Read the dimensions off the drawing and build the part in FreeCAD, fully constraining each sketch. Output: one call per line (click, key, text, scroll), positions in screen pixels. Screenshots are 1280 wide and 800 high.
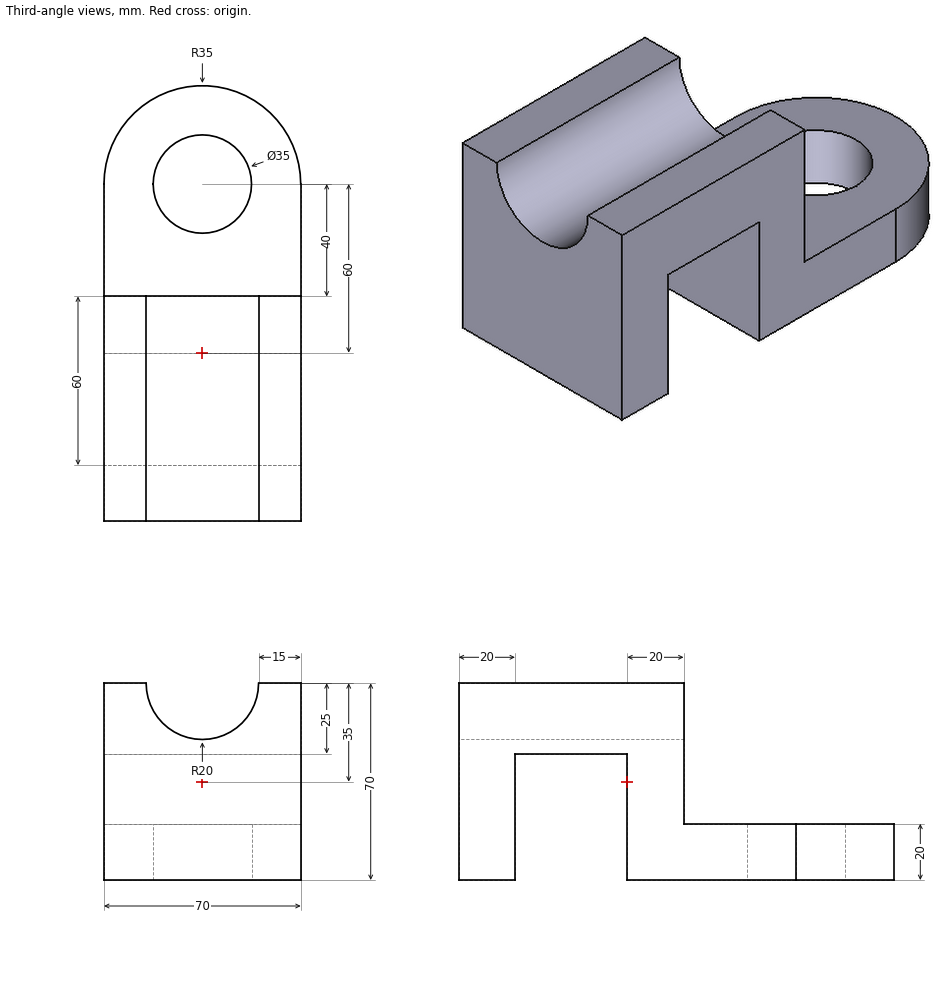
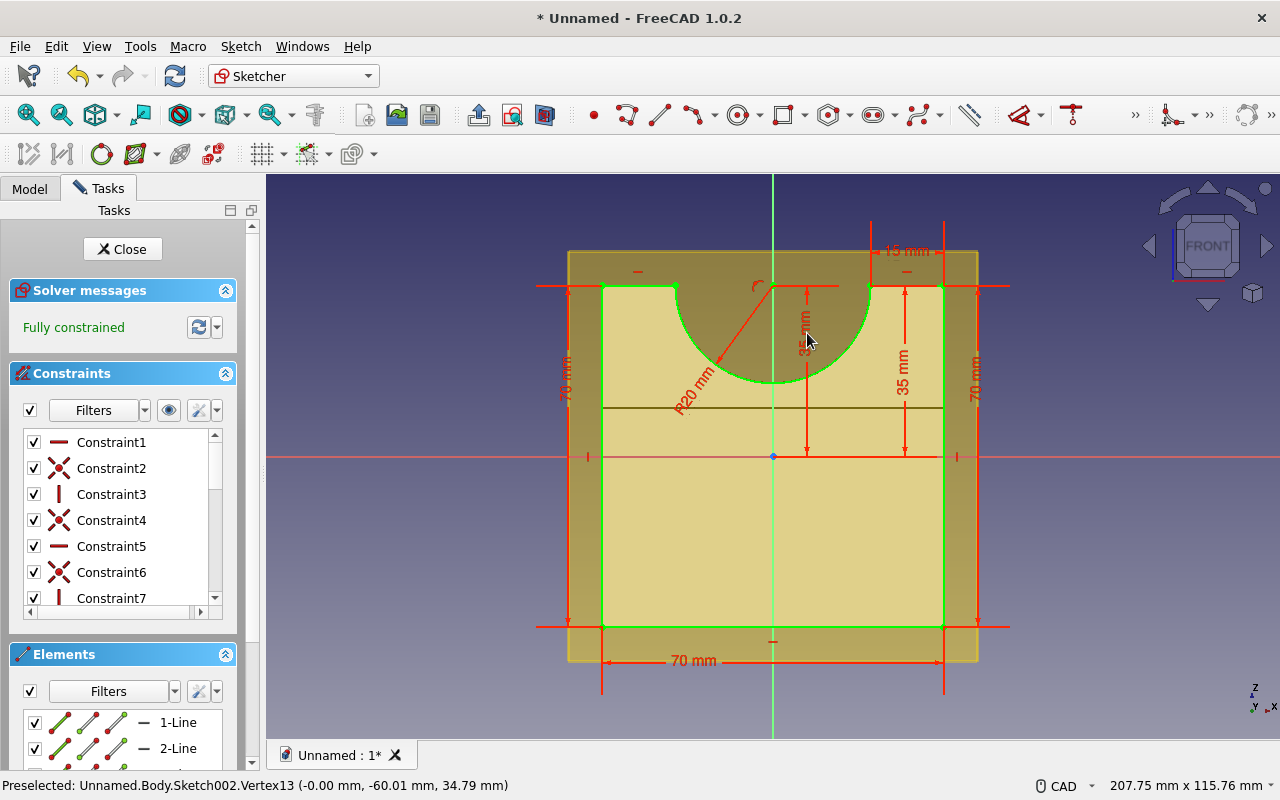
click(123, 249)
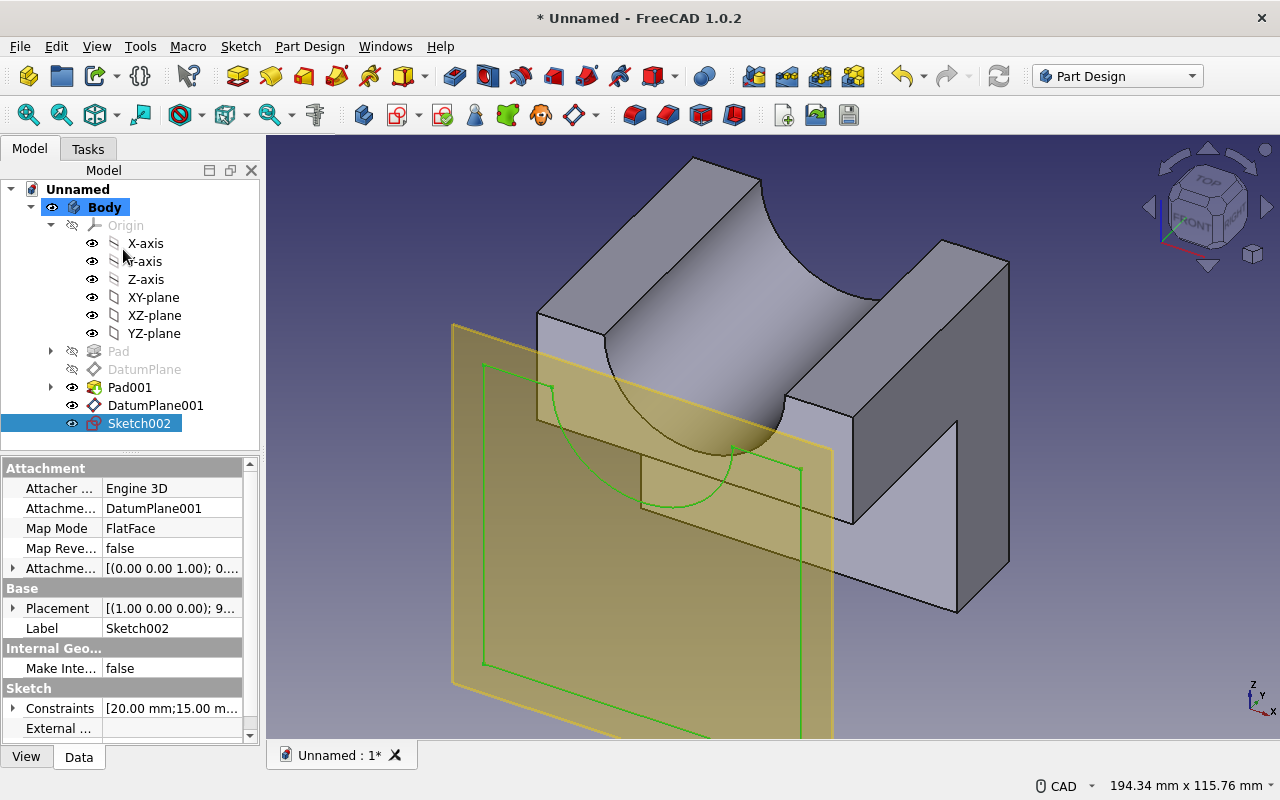
click(238, 76)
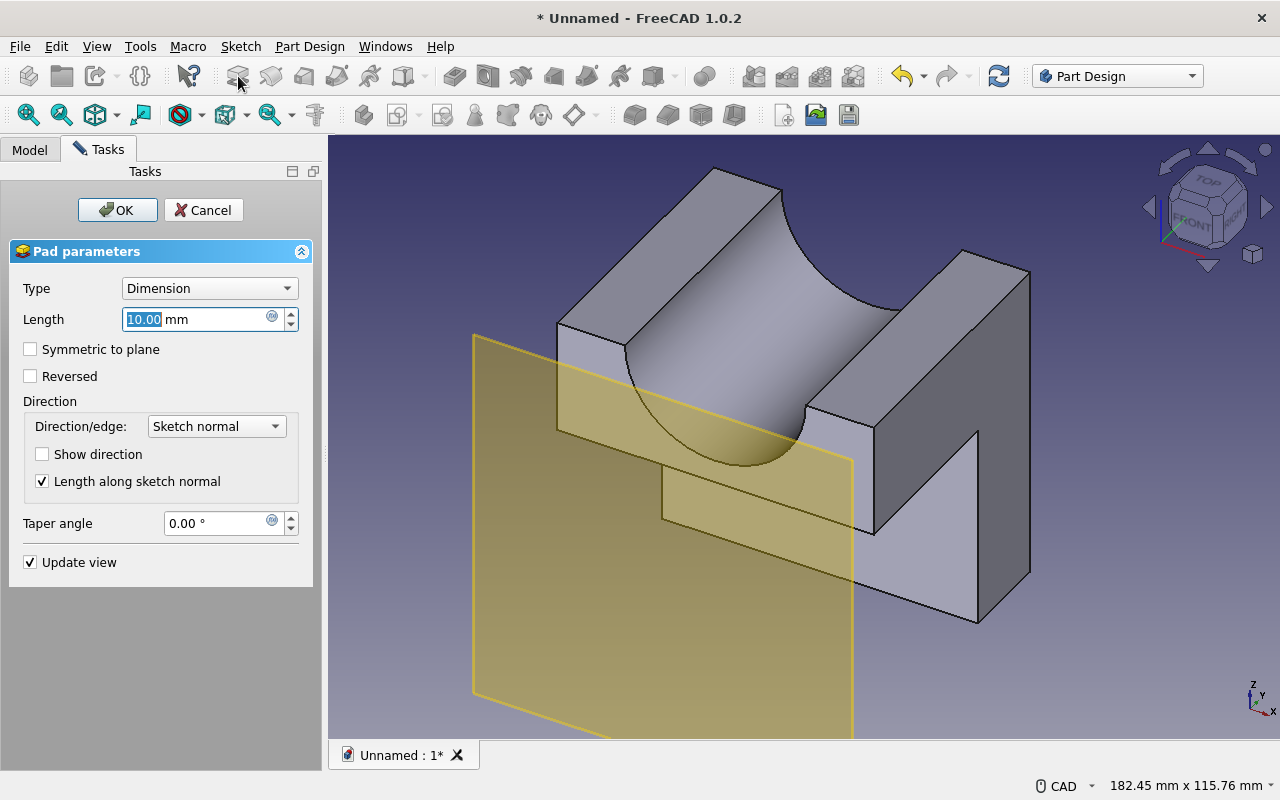
text(20)
key(Tab)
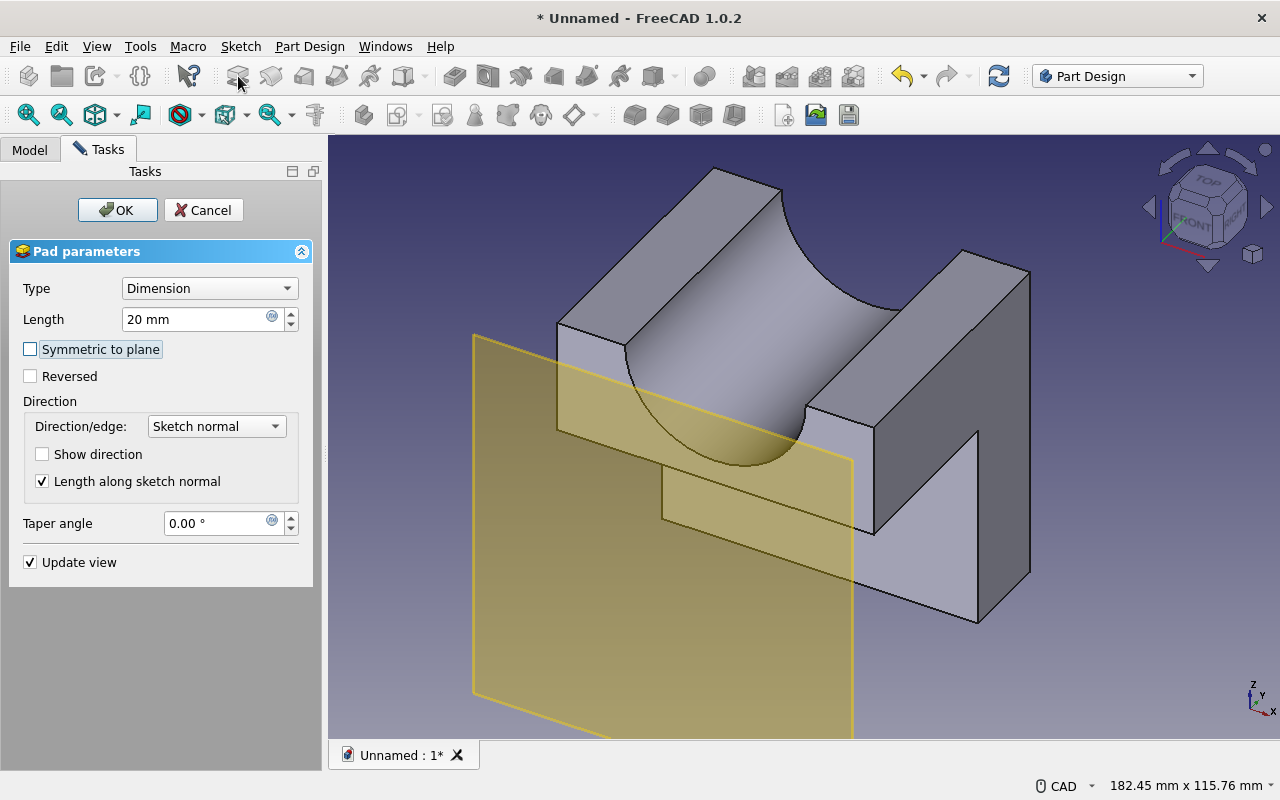
click(31, 376)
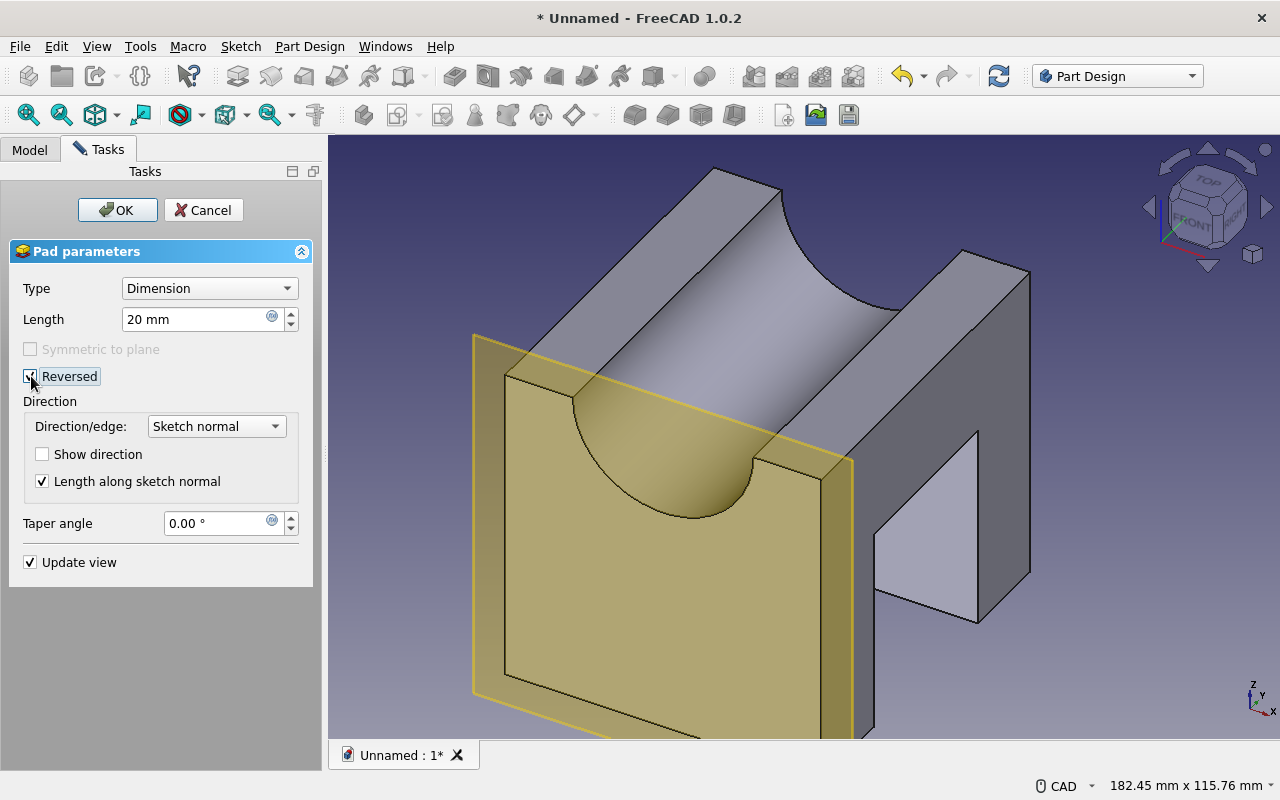
click(118, 210)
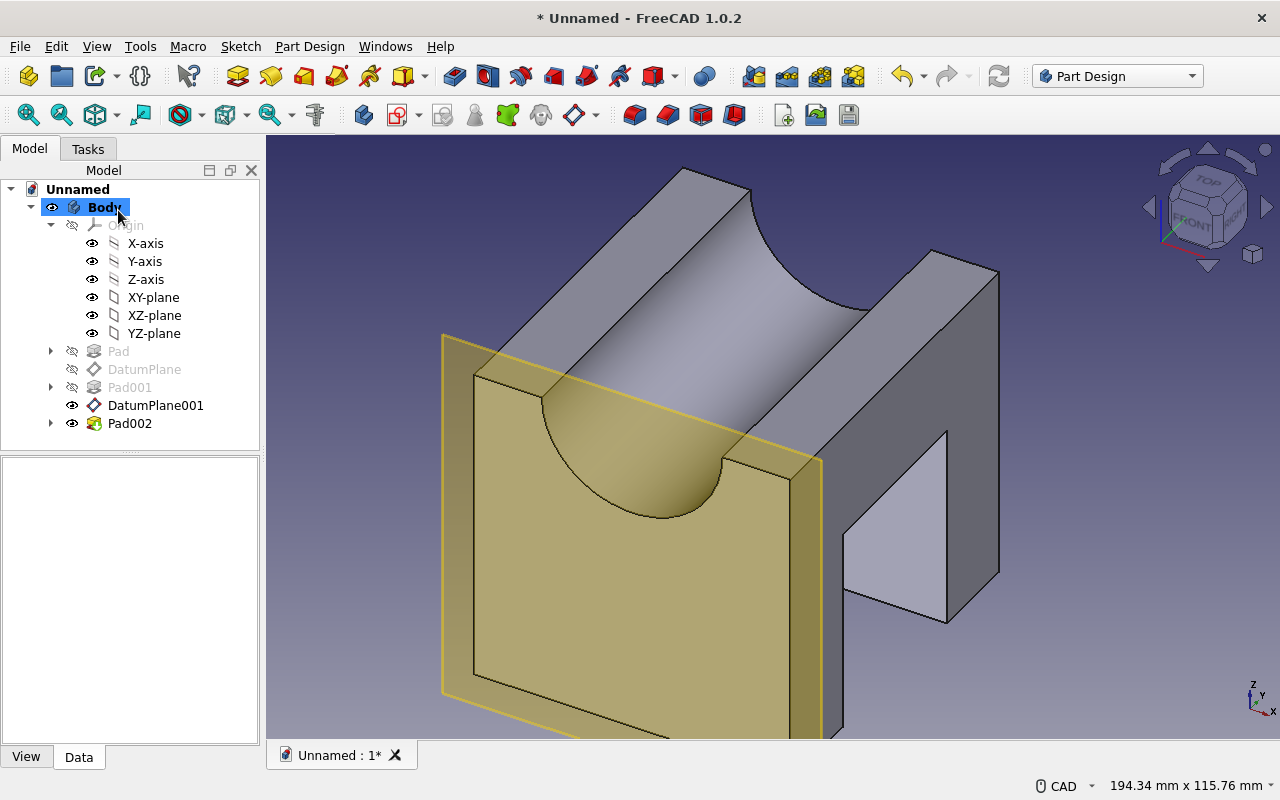
click(117, 405)
key(space)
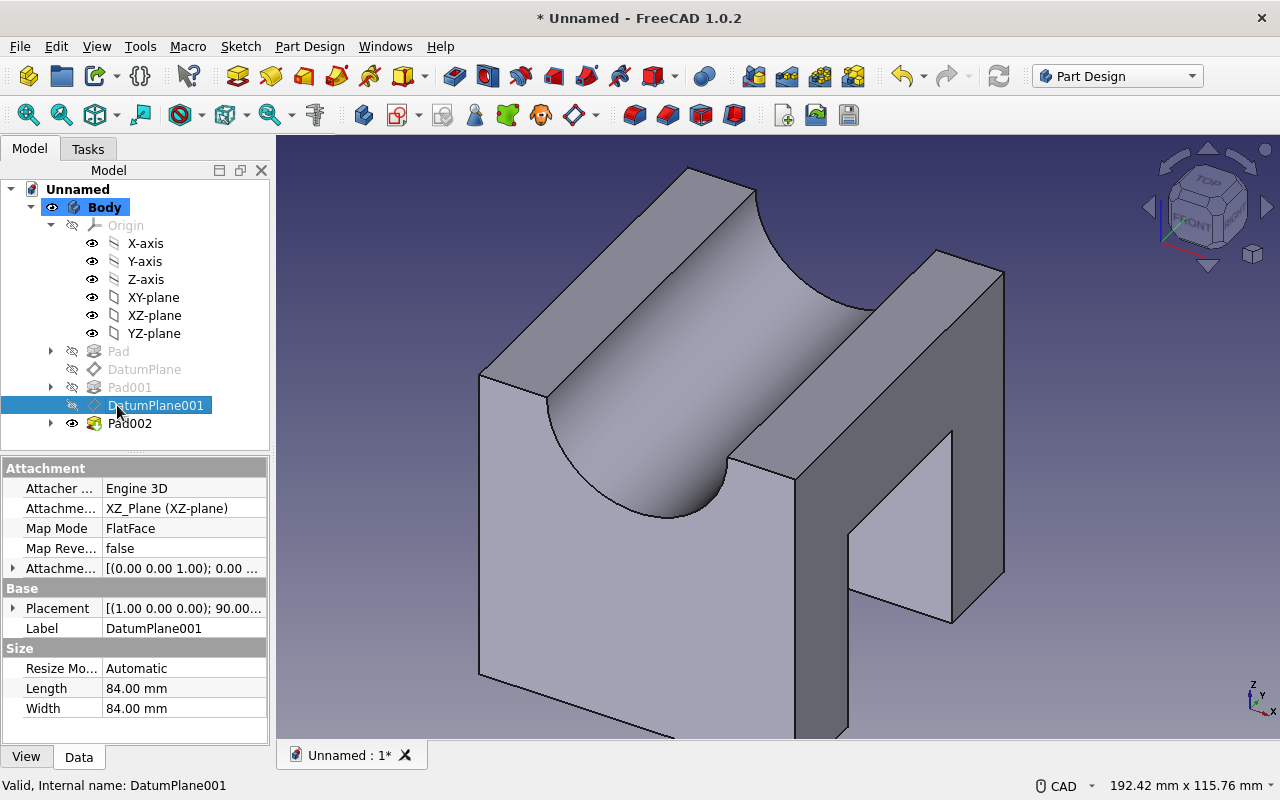
click(29, 116)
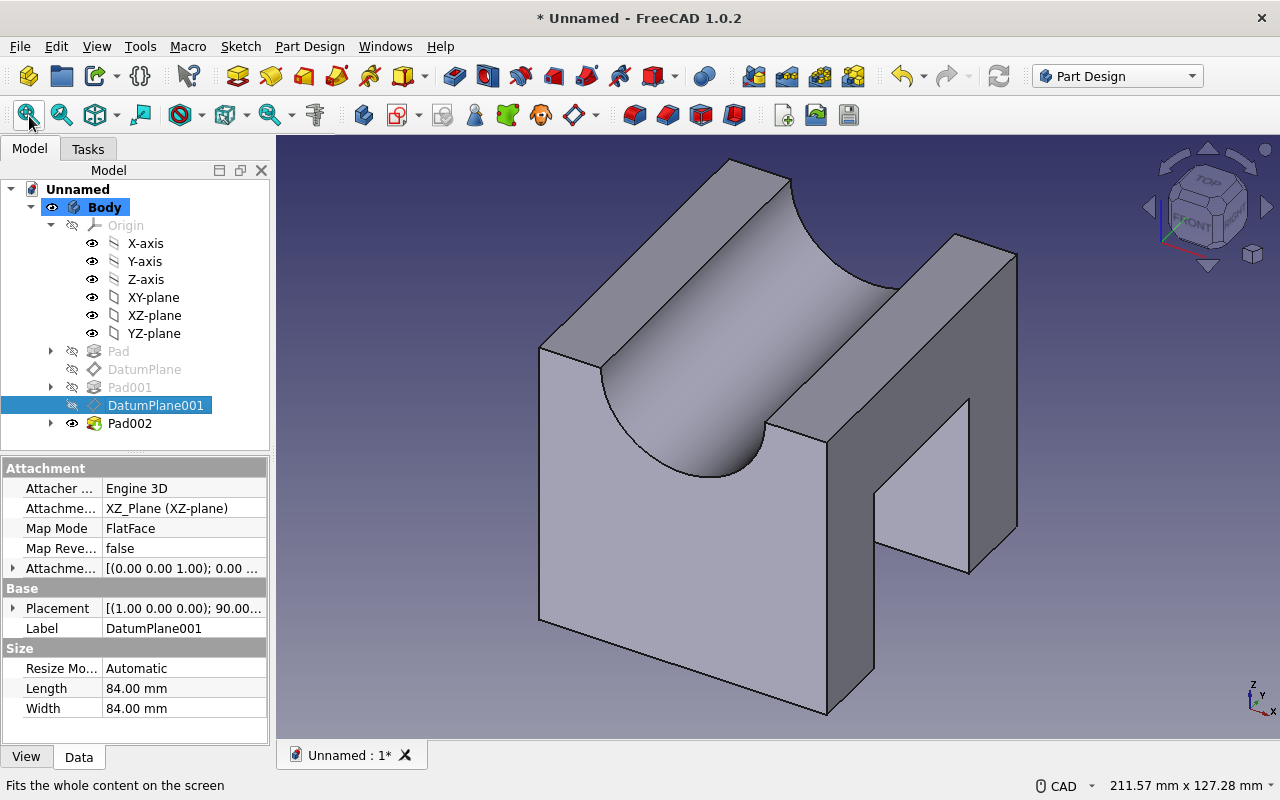
key(5)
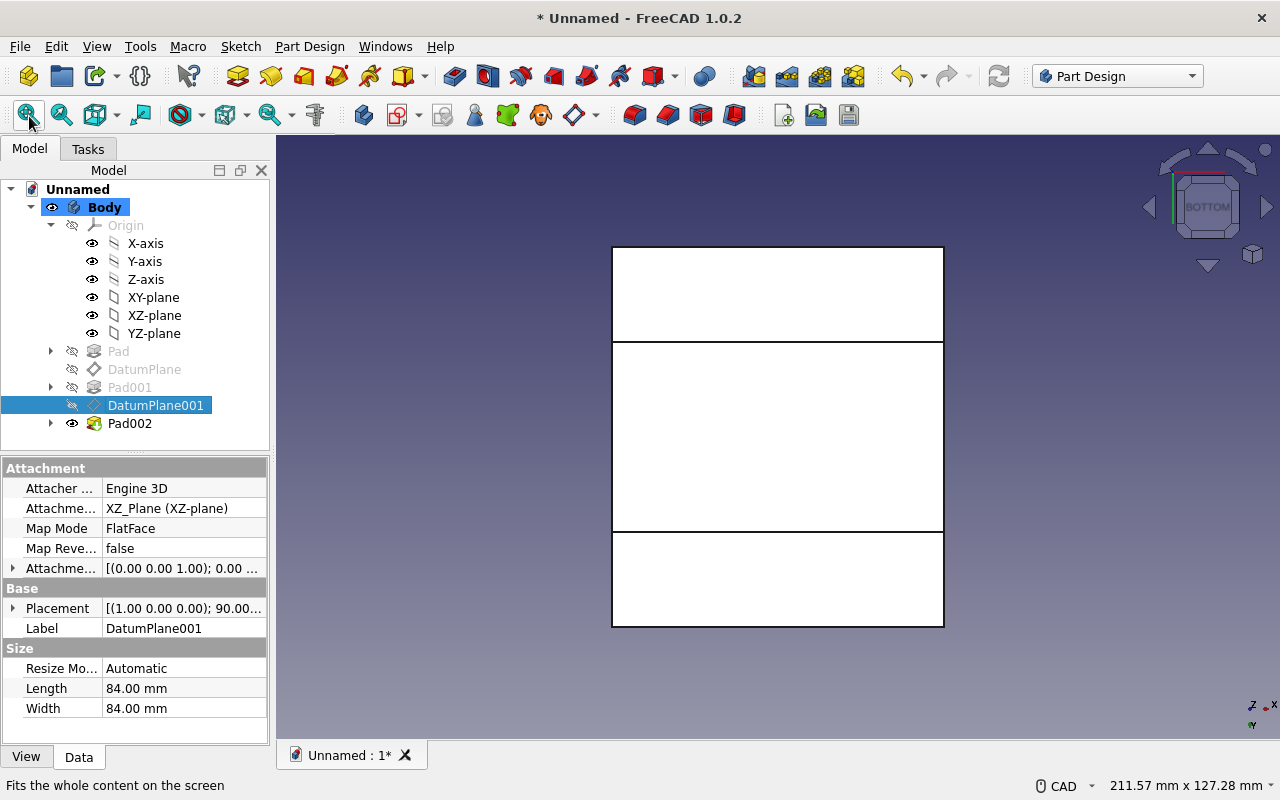
click(873, 578)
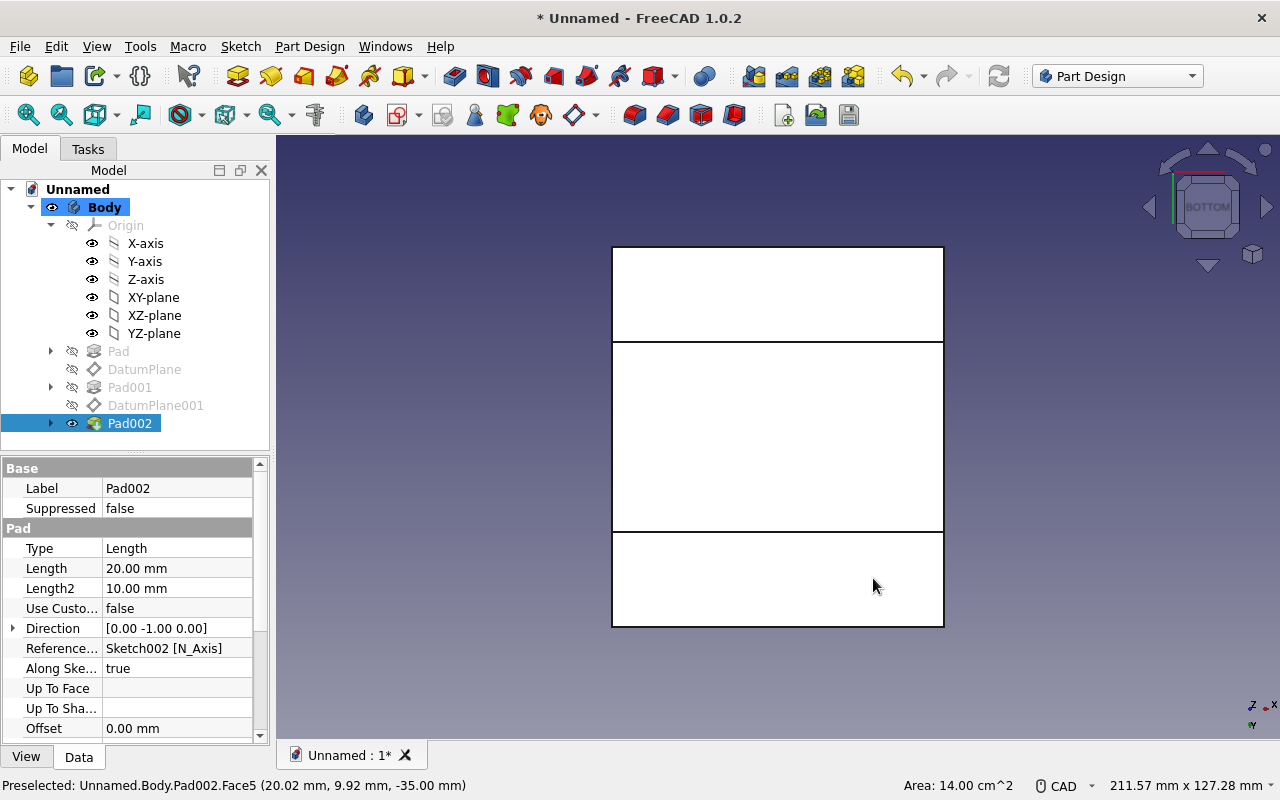
click(396, 116)